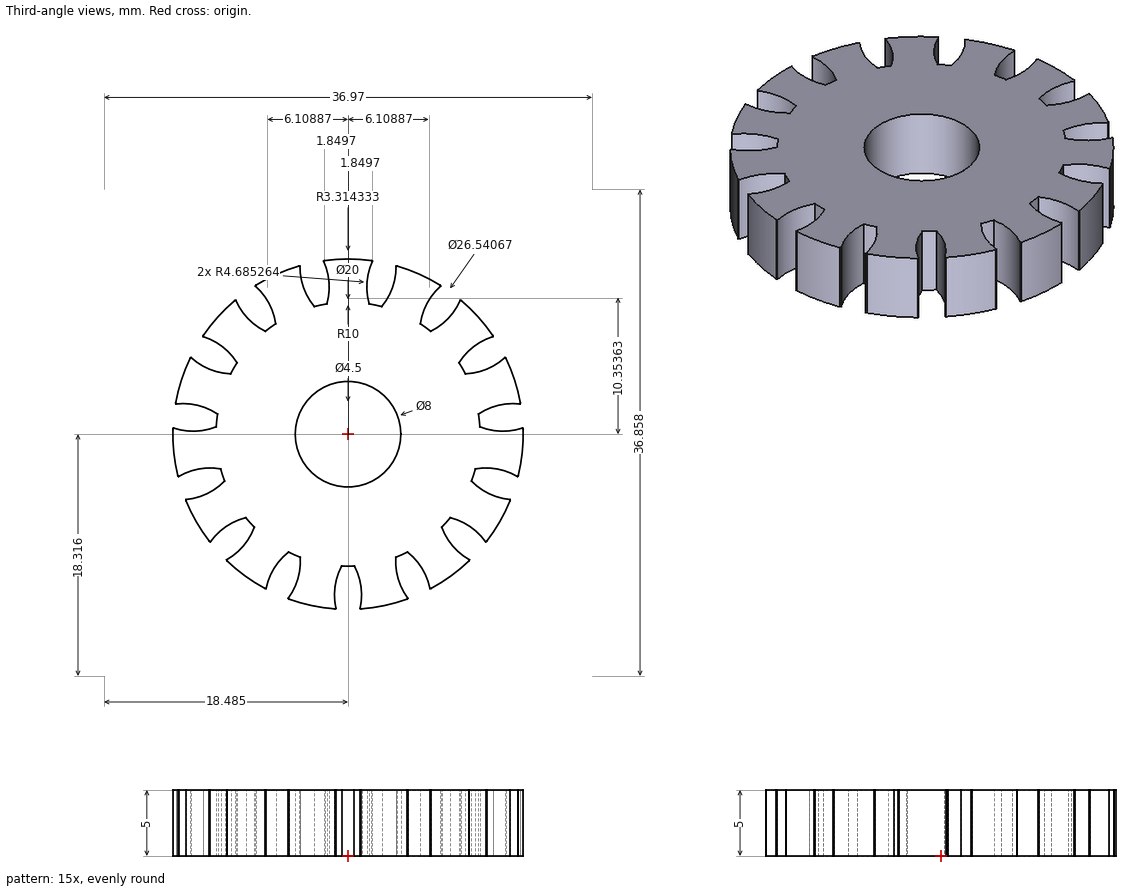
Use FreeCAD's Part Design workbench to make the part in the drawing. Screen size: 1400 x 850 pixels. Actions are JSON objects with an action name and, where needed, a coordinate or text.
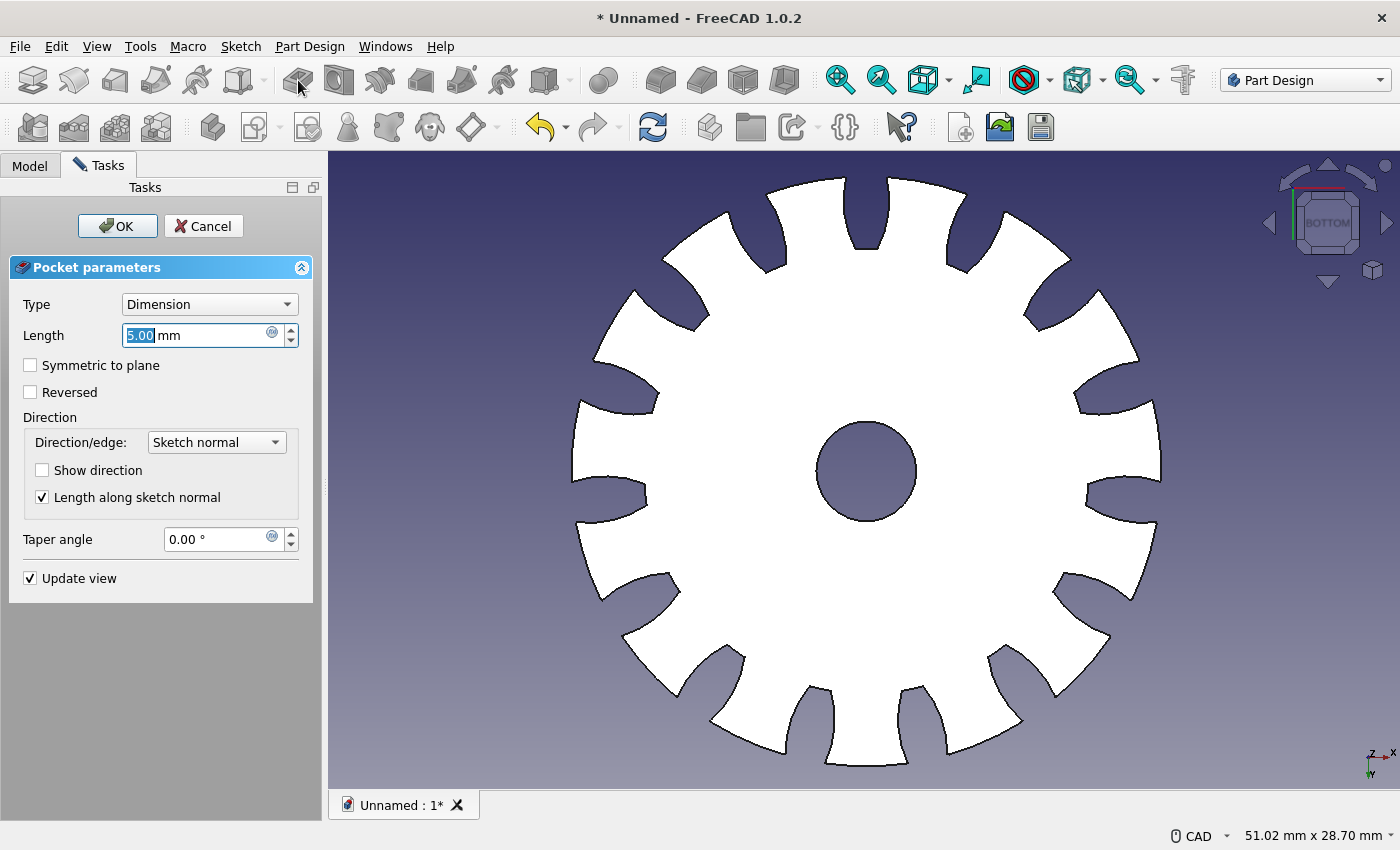
{"action": "left_click", "coordinate": [210, 304]}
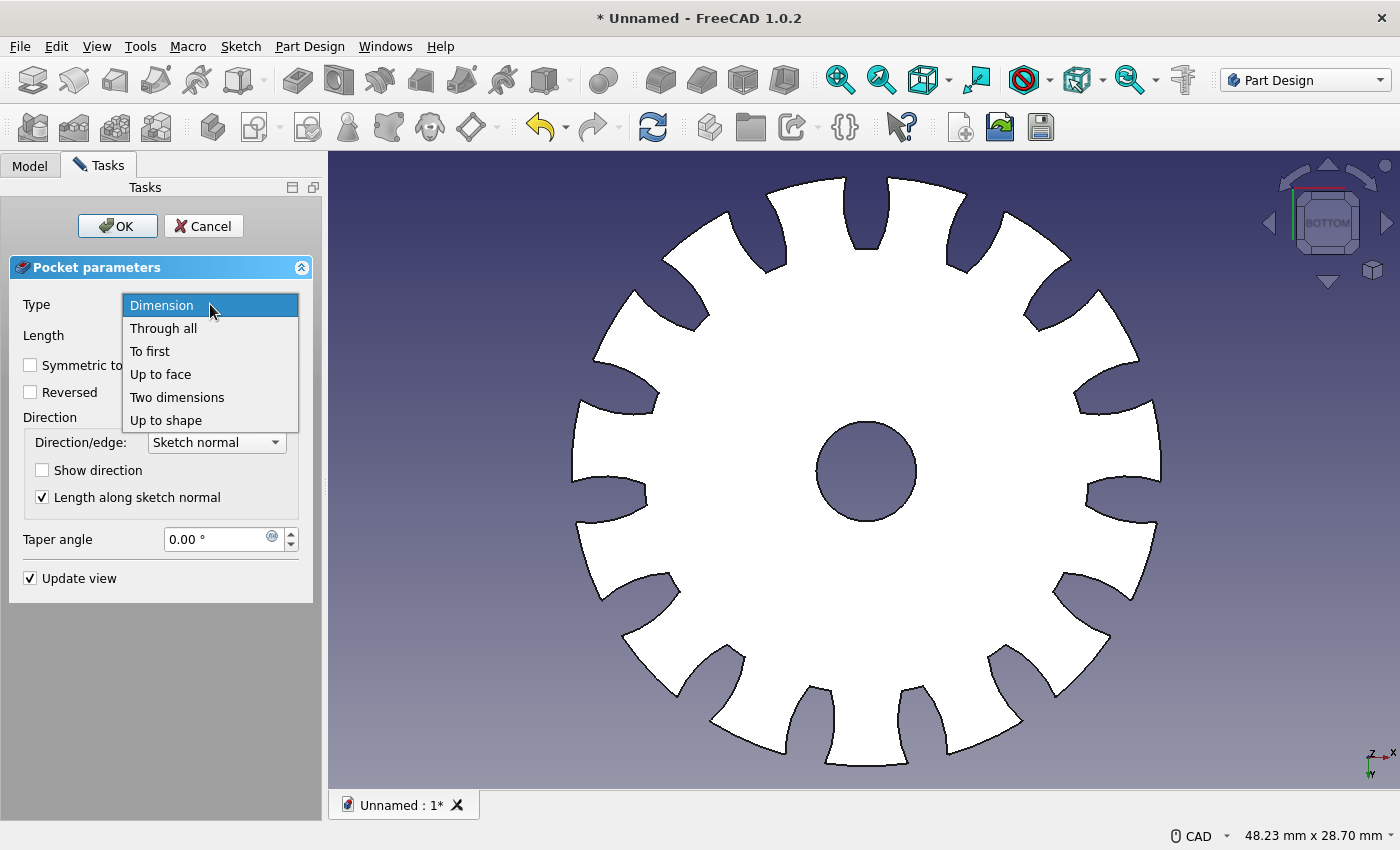
{"action": "left_click", "coordinate": [208, 328]}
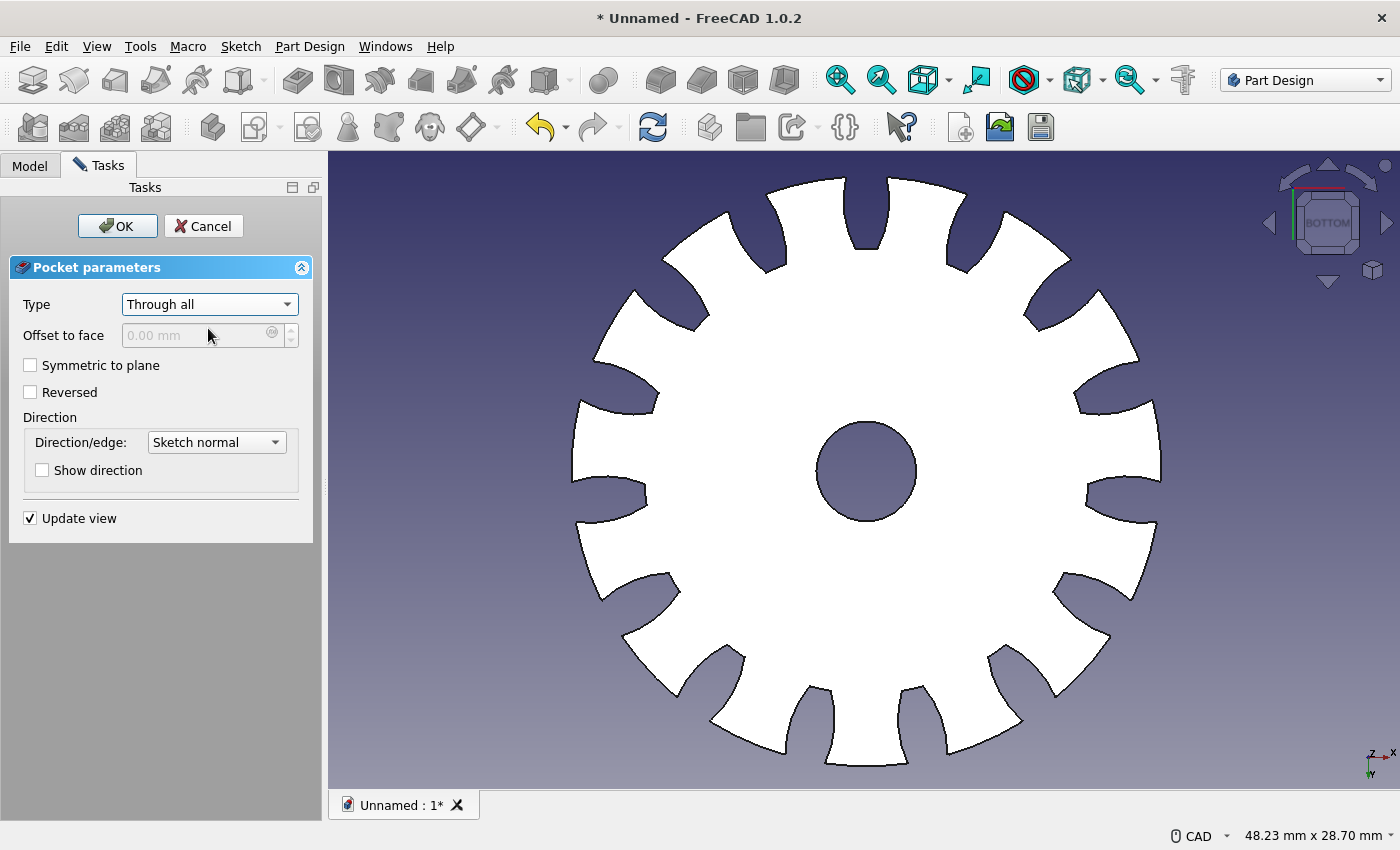
{"action": "left_click", "coordinate": [118, 226]}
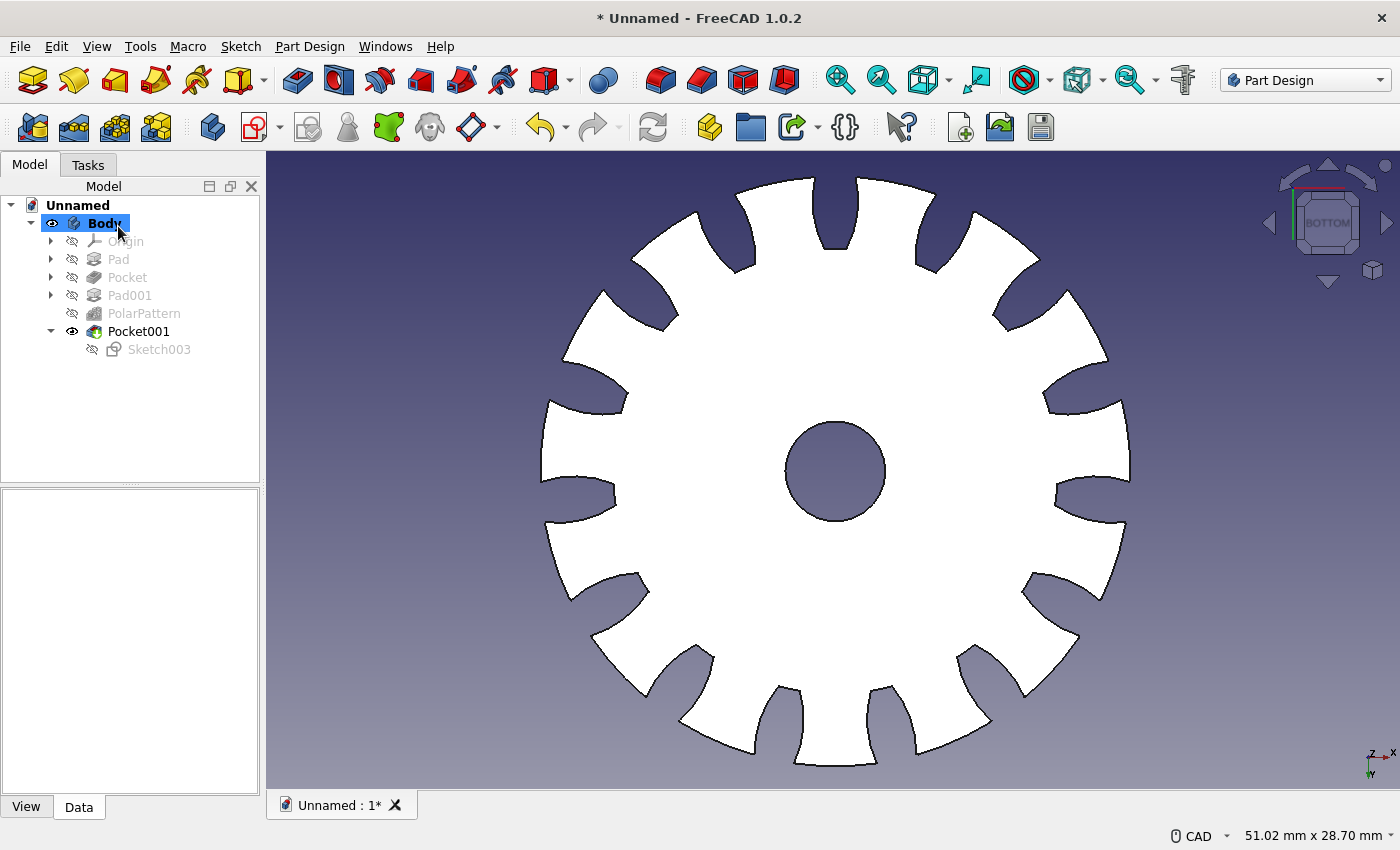
{"action": "key", "text": "0"}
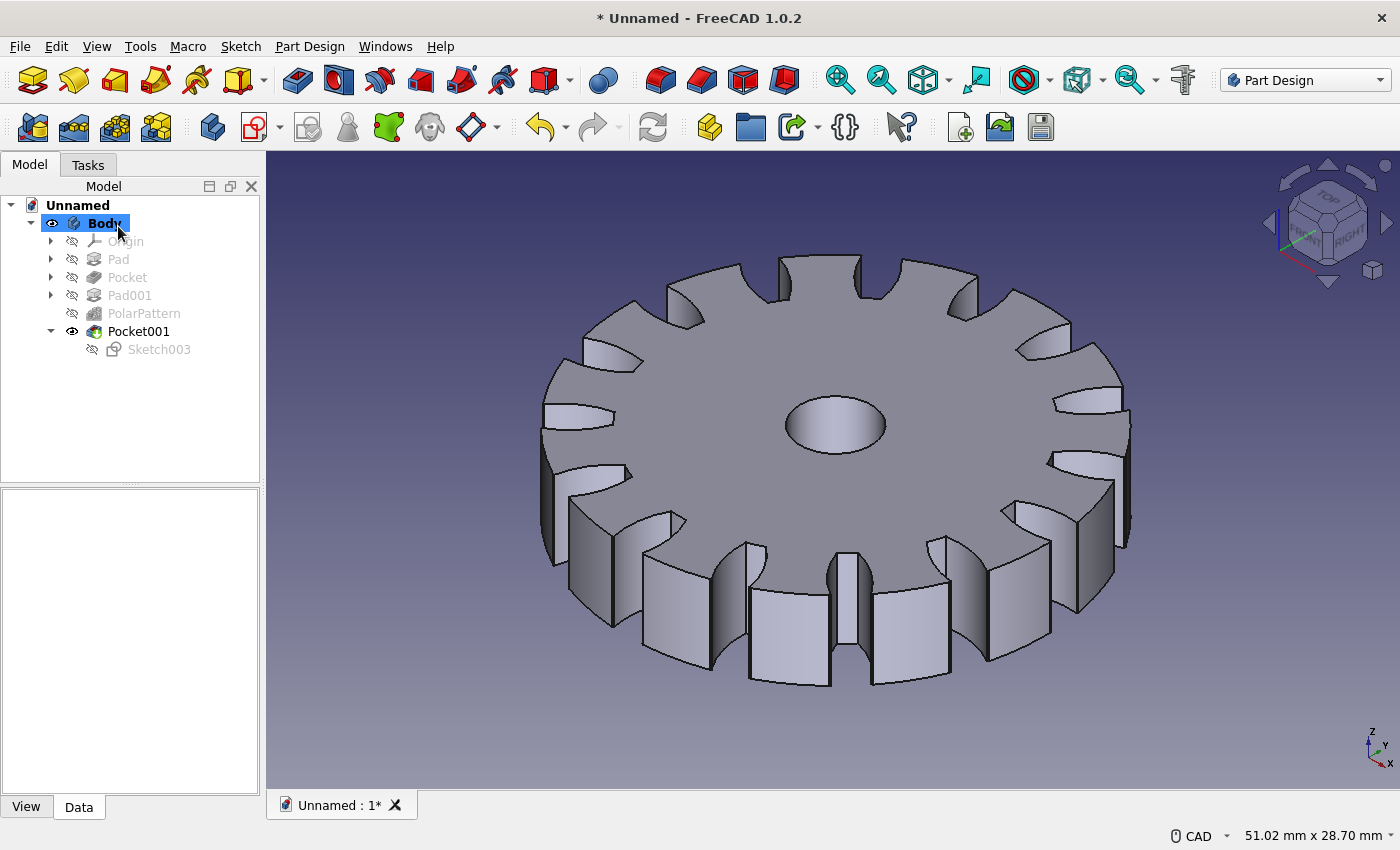
{"action": "left_click", "coordinate": [836, 355]}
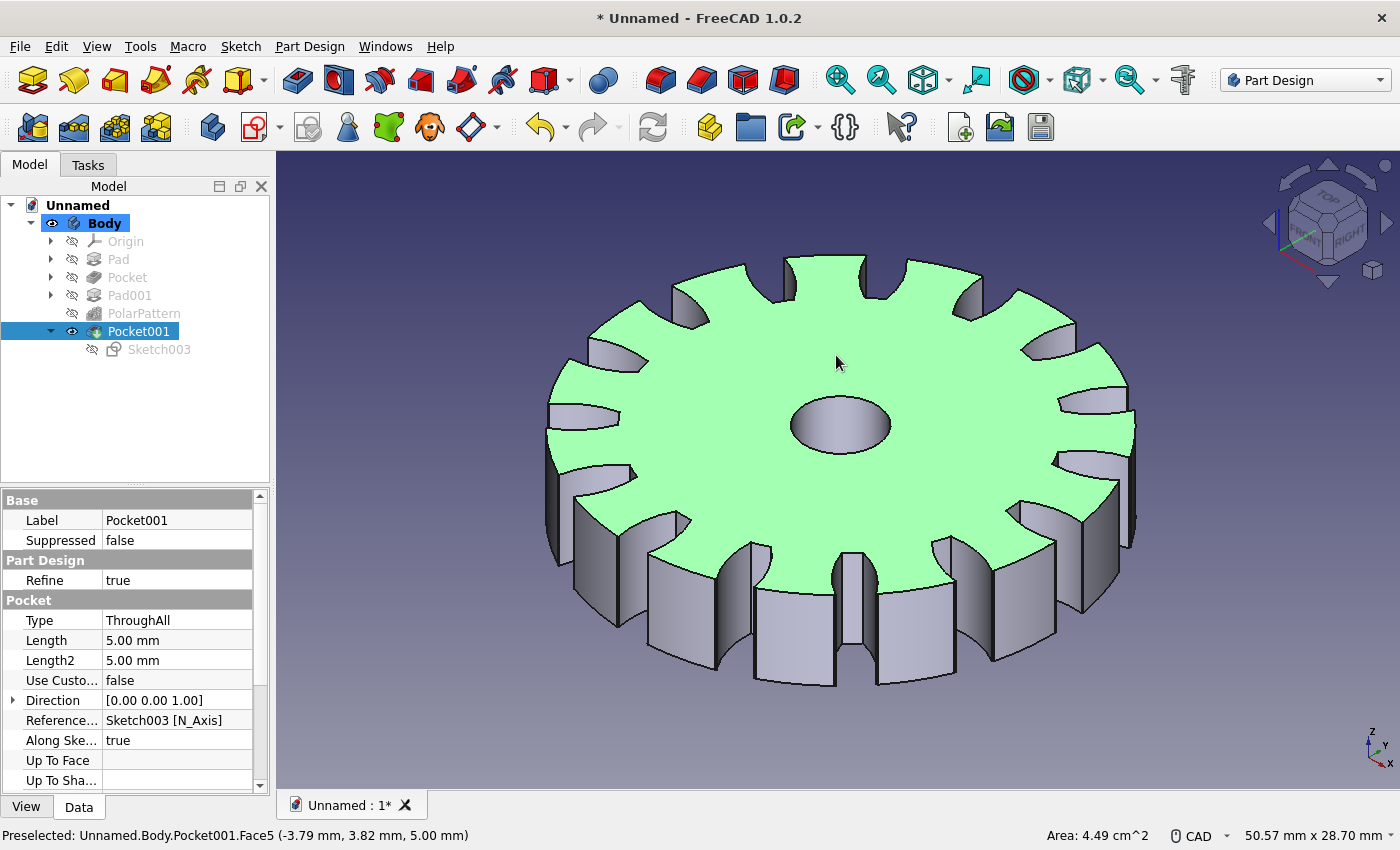
{"action": "left_click", "coordinate": [254, 128]}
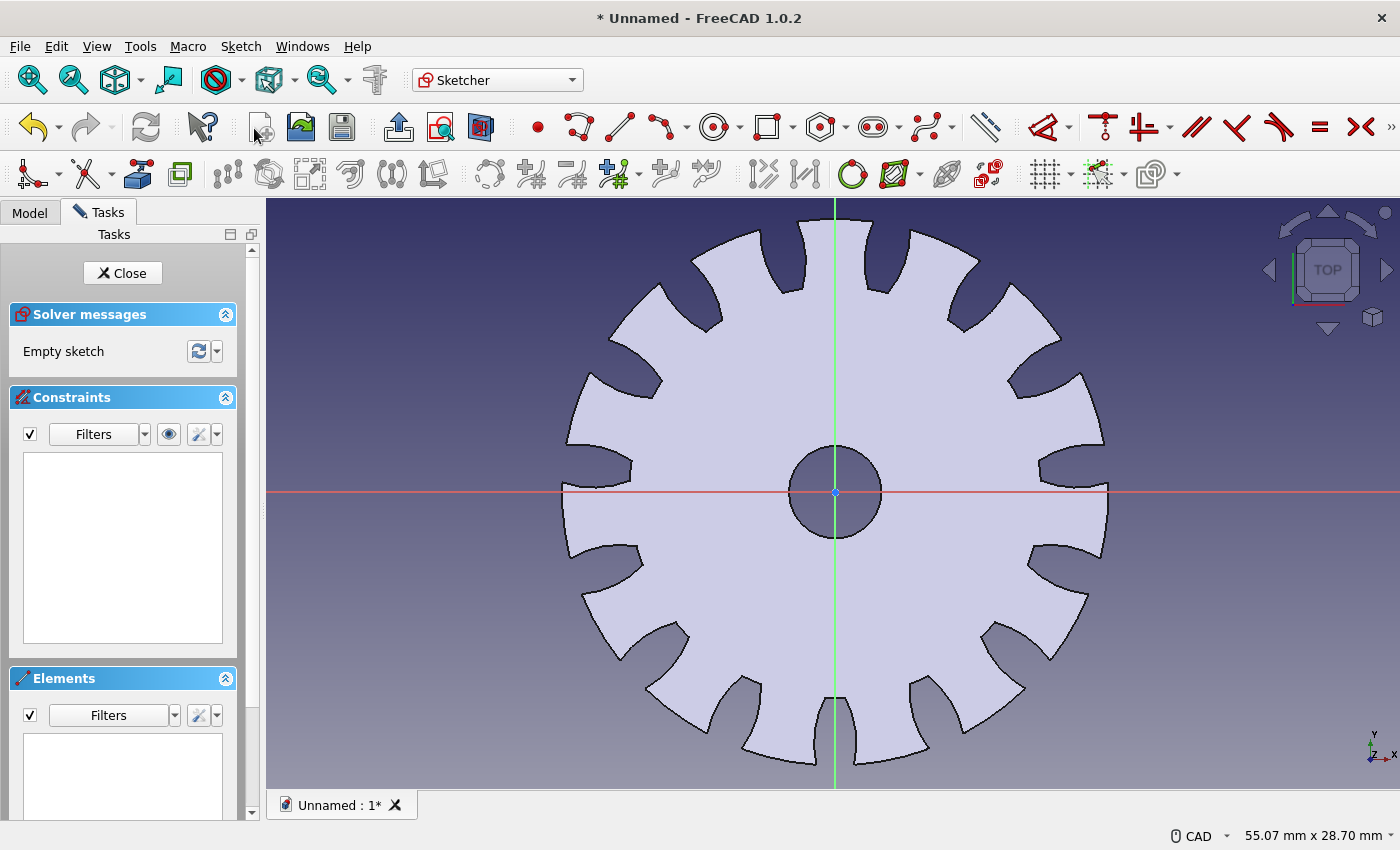
{"action": "scroll", "coordinate": [893, 491], "scroll_direction": "up", "scroll_amount": 4}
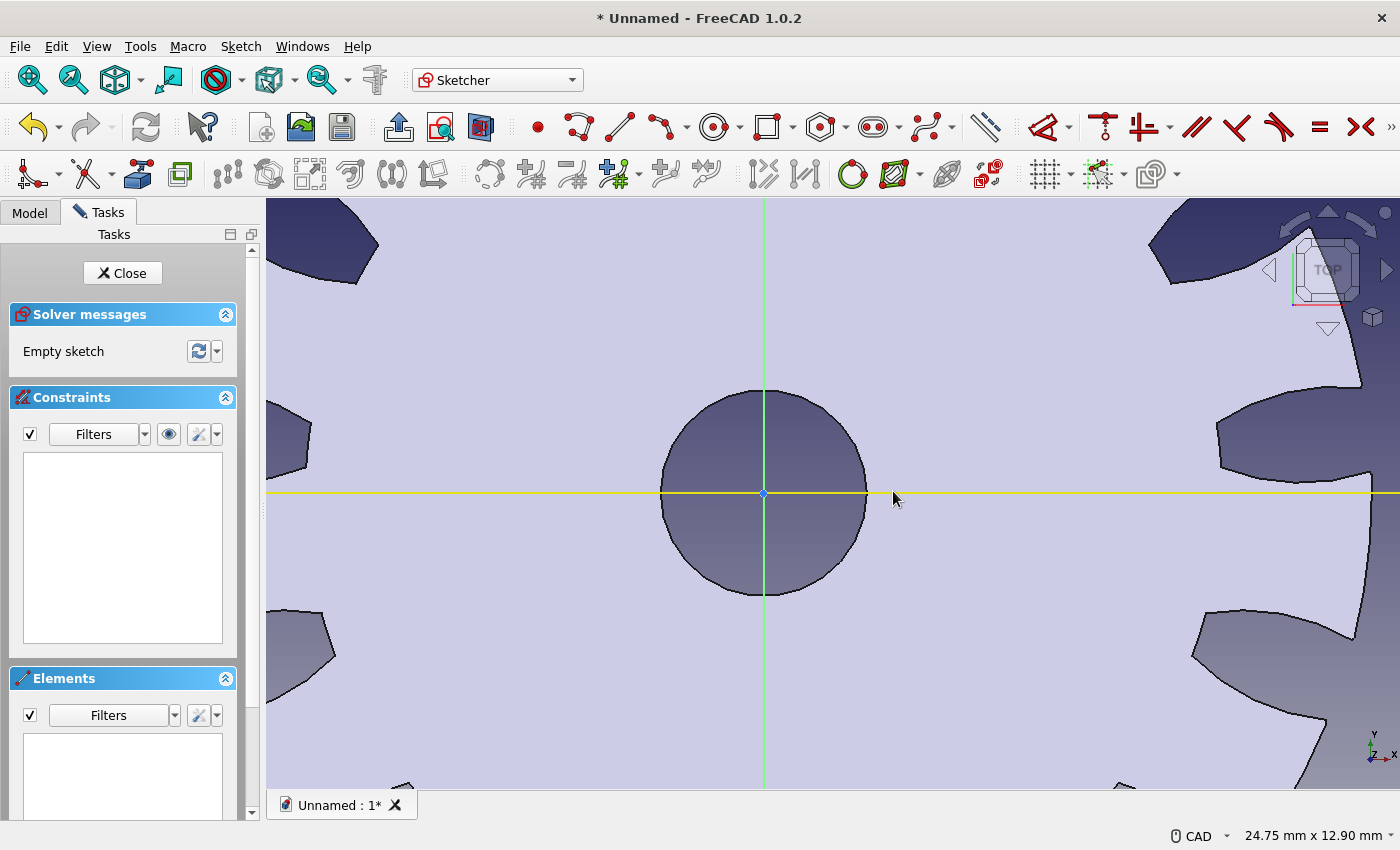
{"action": "left_click", "coordinate": [714, 128]}